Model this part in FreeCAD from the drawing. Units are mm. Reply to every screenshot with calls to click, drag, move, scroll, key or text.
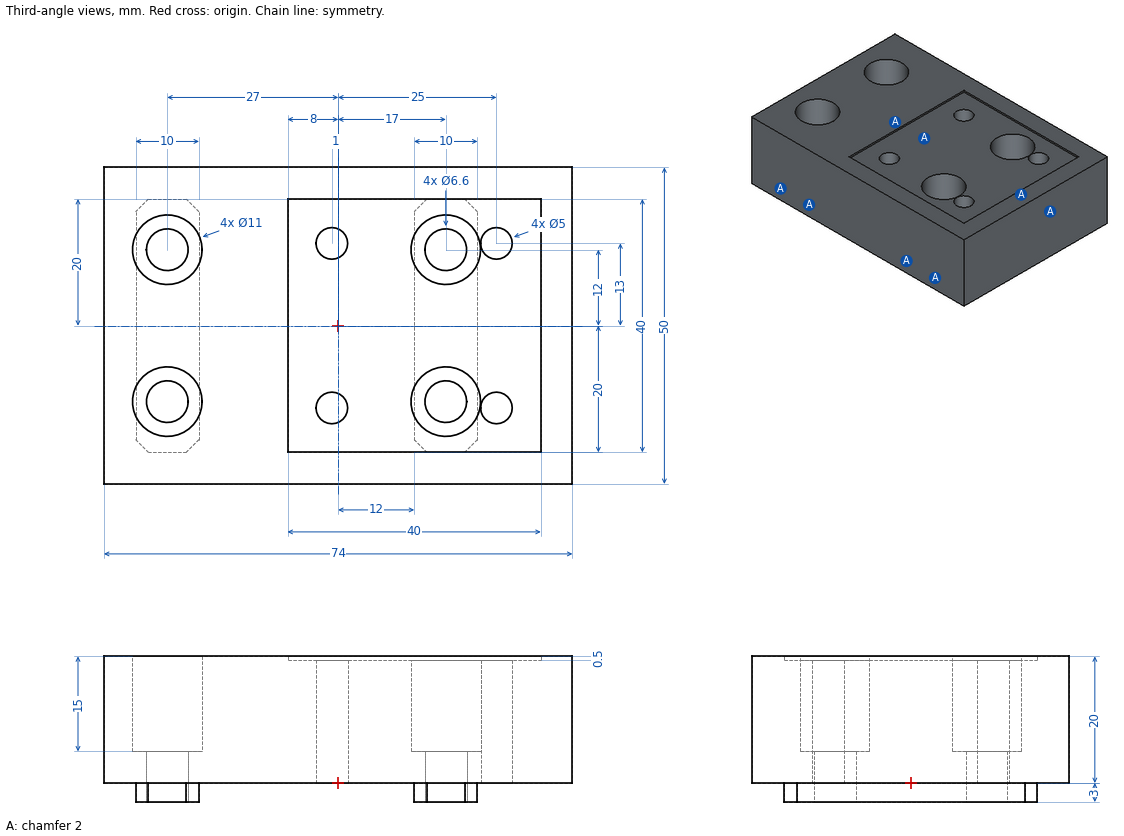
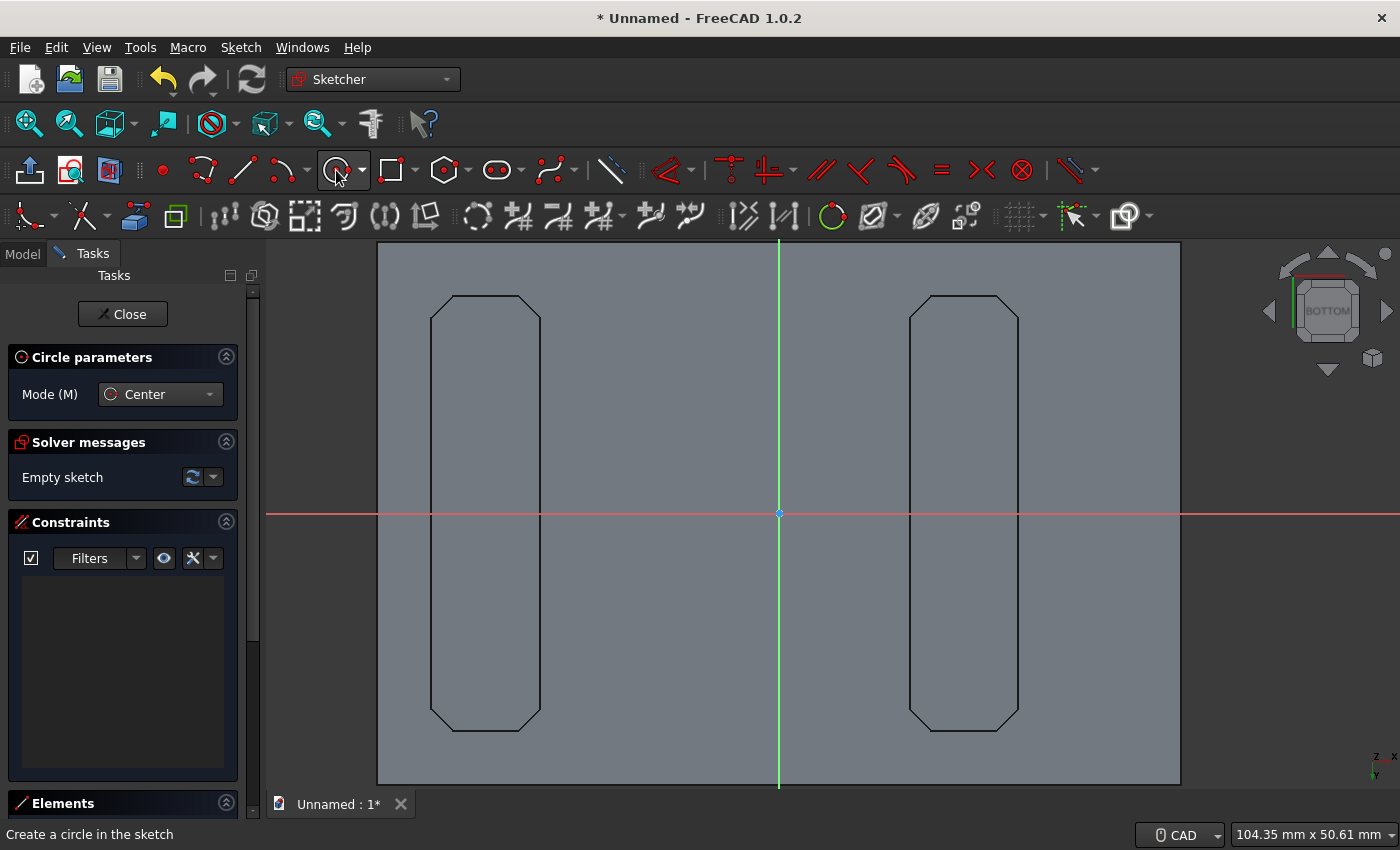
click(964, 644)
move(989, 619)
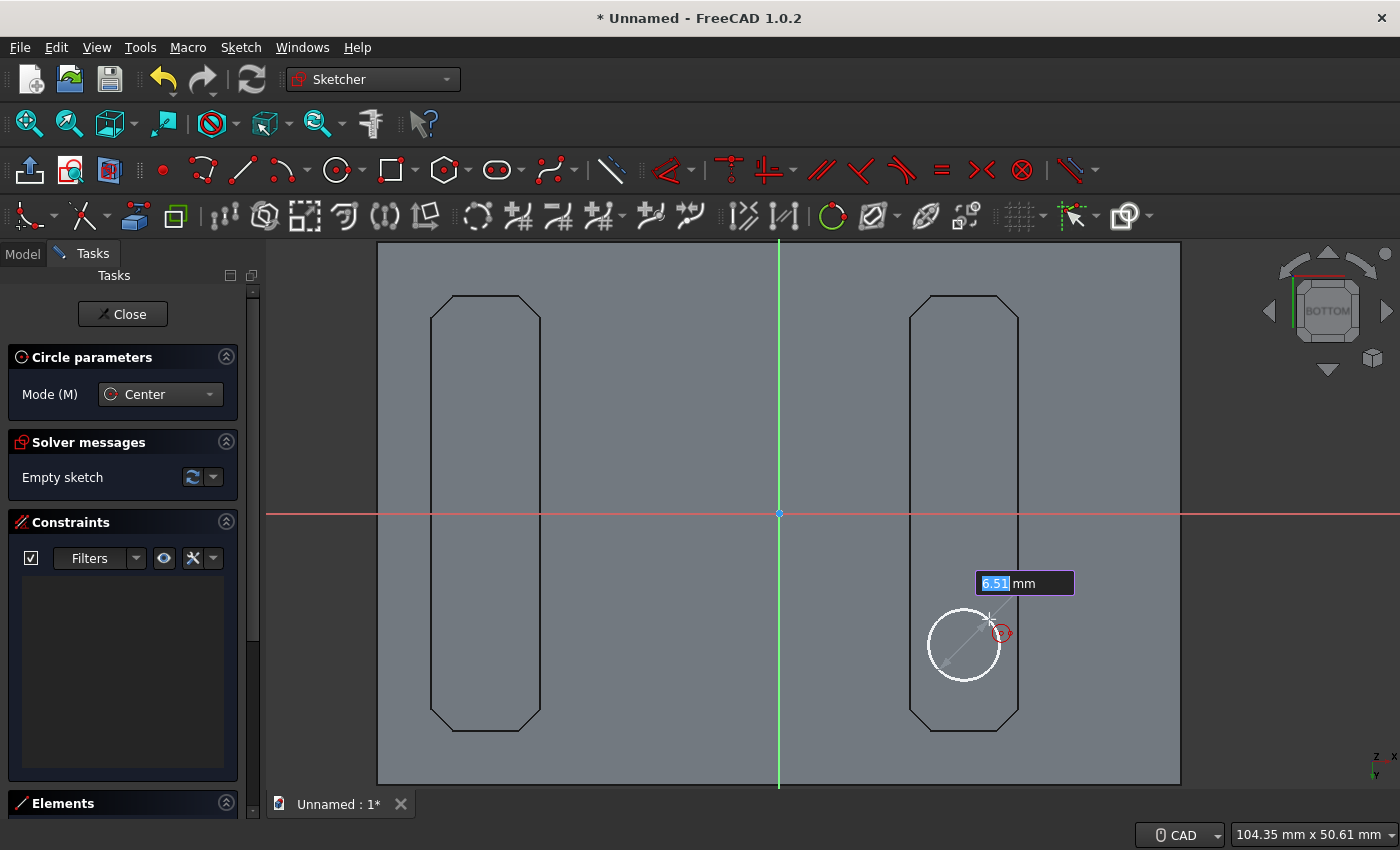
text(6.6)
key(Return)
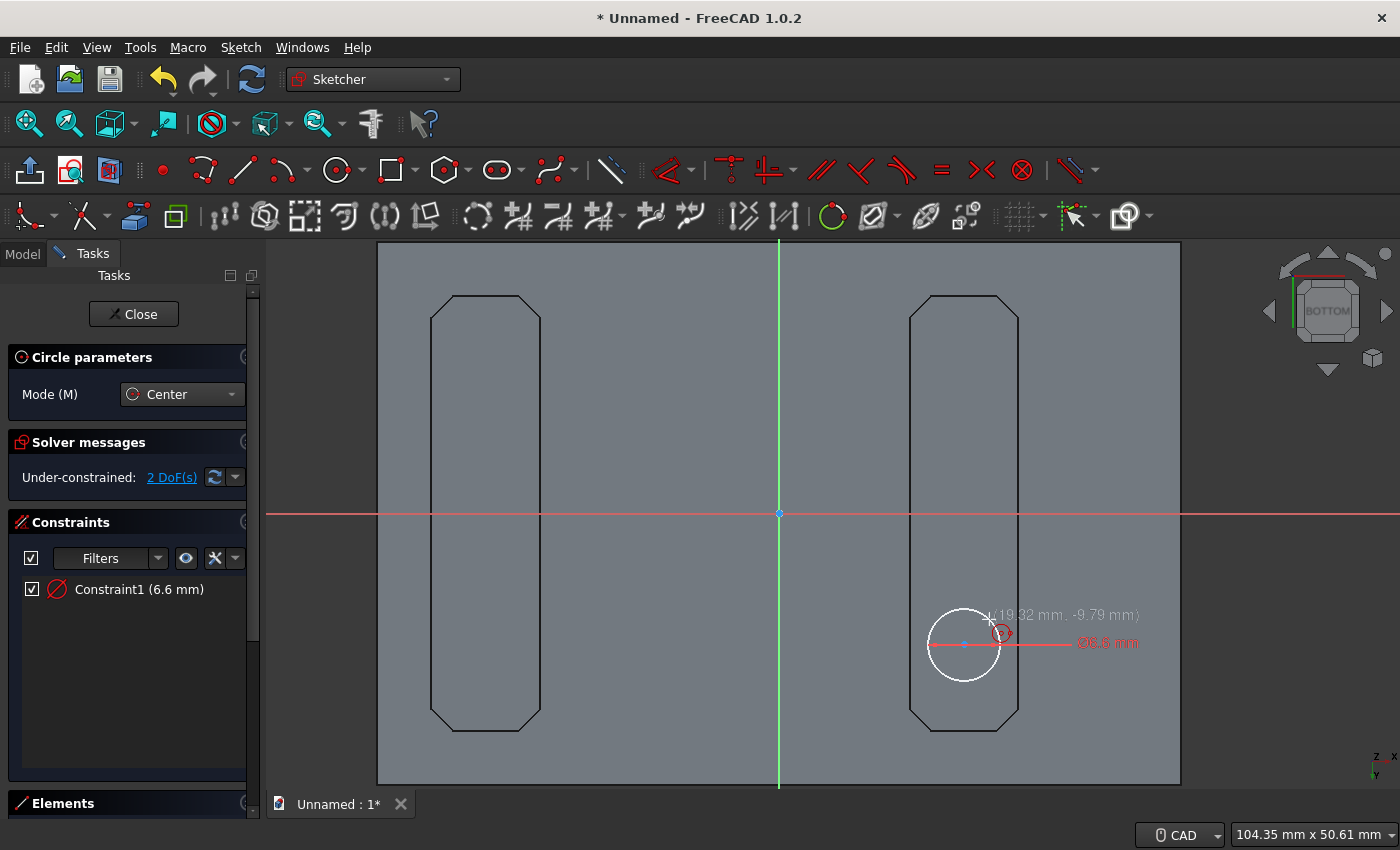
click(486, 644)
move(511, 619)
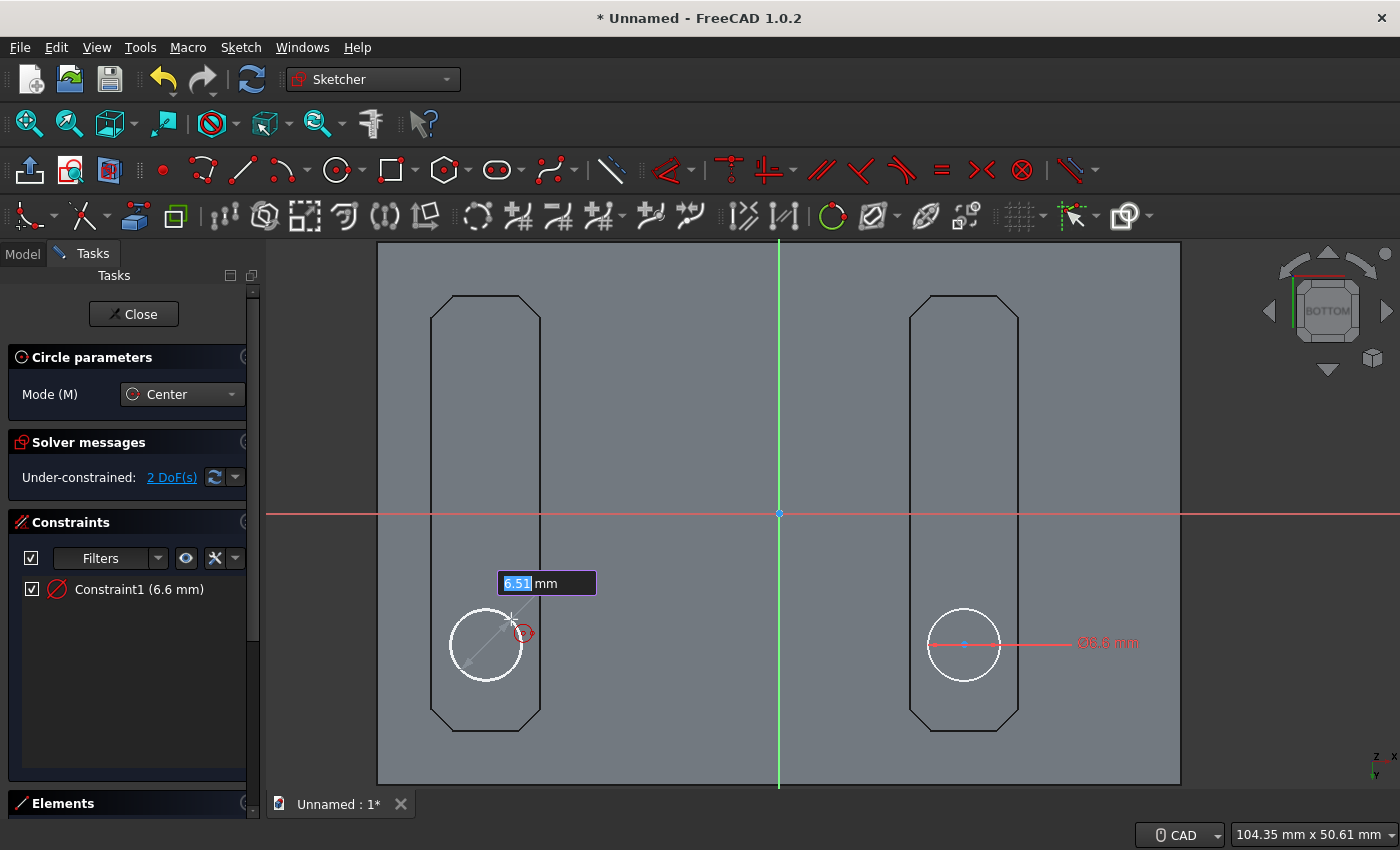
text(6.6)
key(Return)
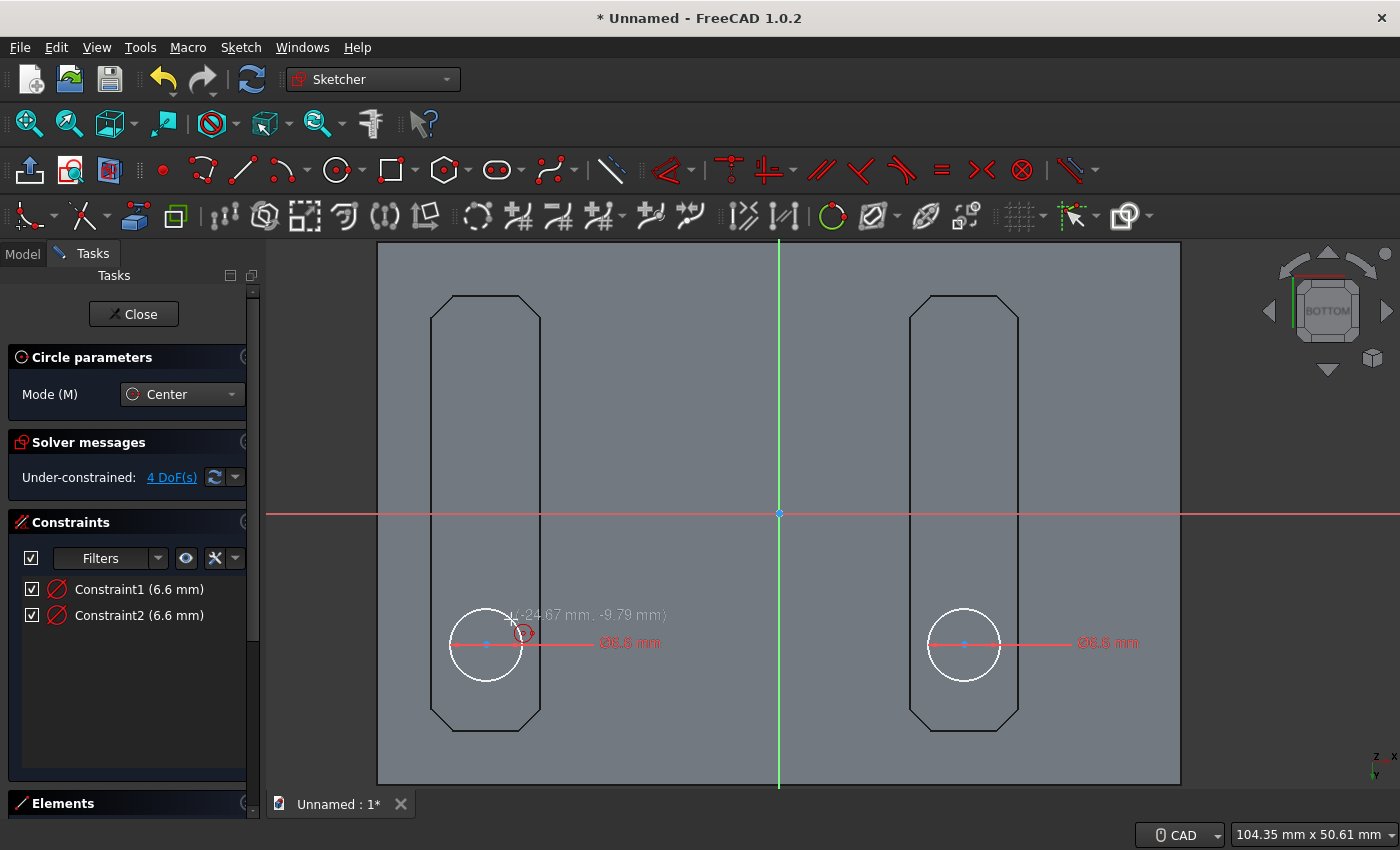
click(1051, 655)
move(1070, 636)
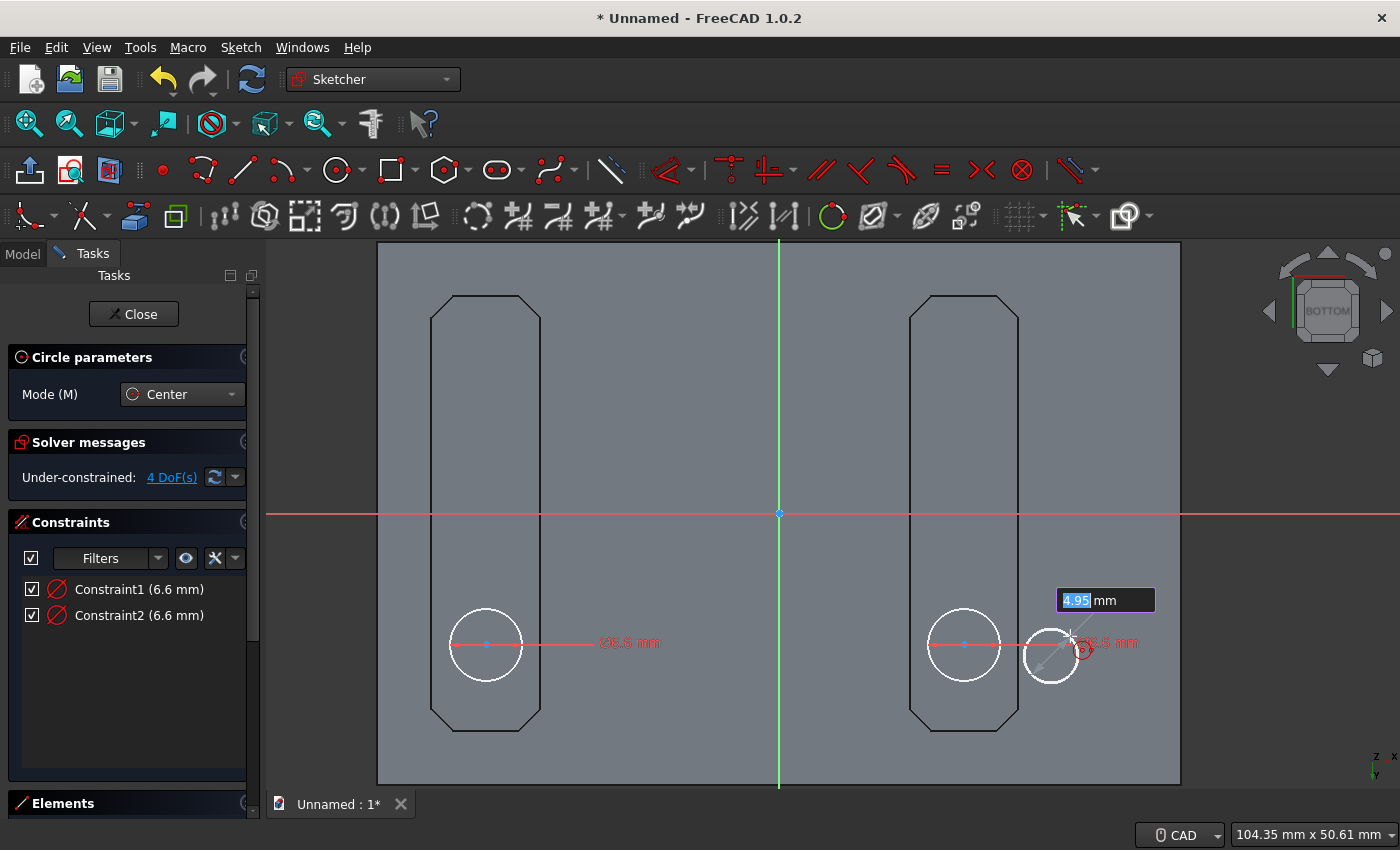
text(5)
key(Return)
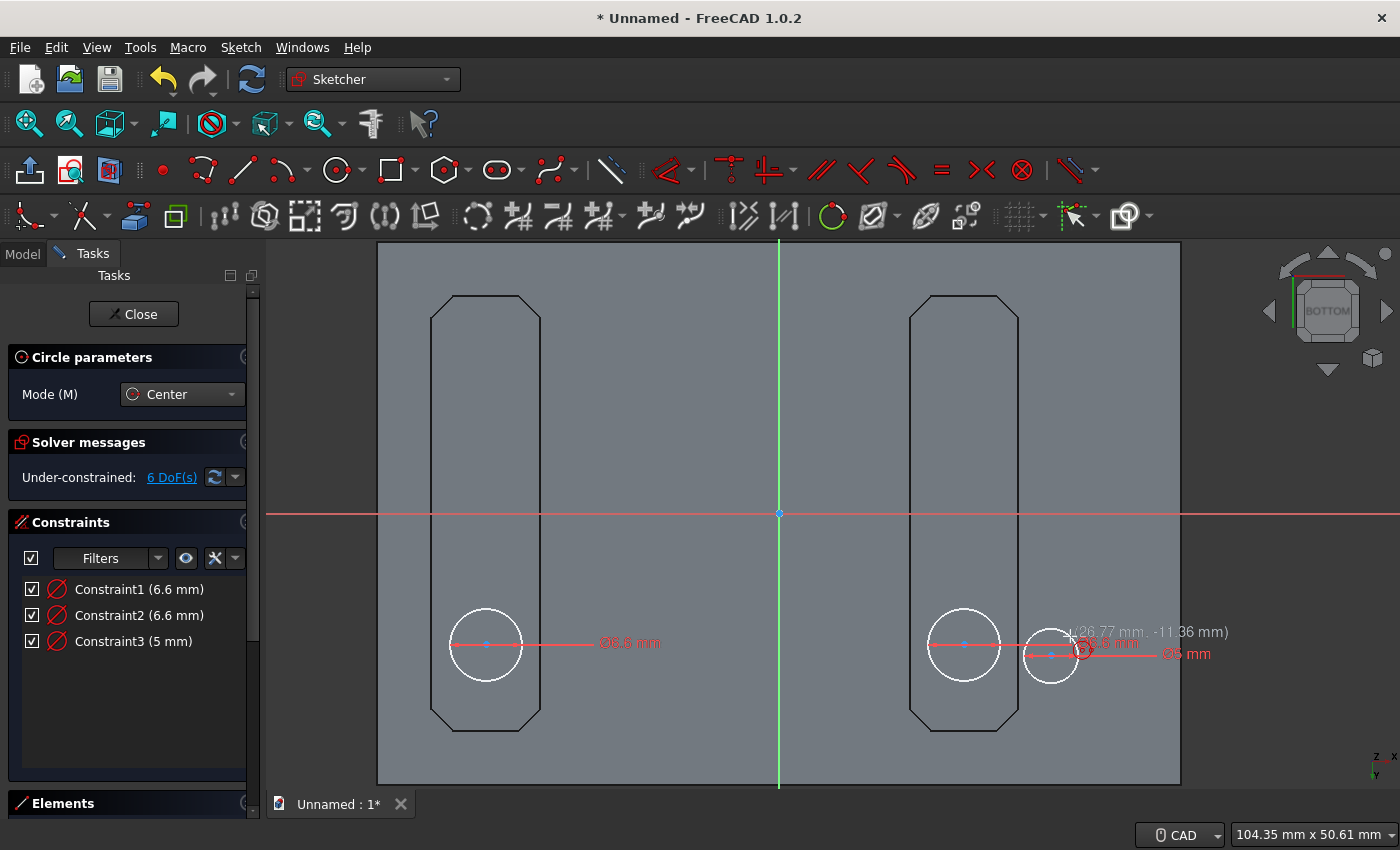
scroll(768, 655, up, 2)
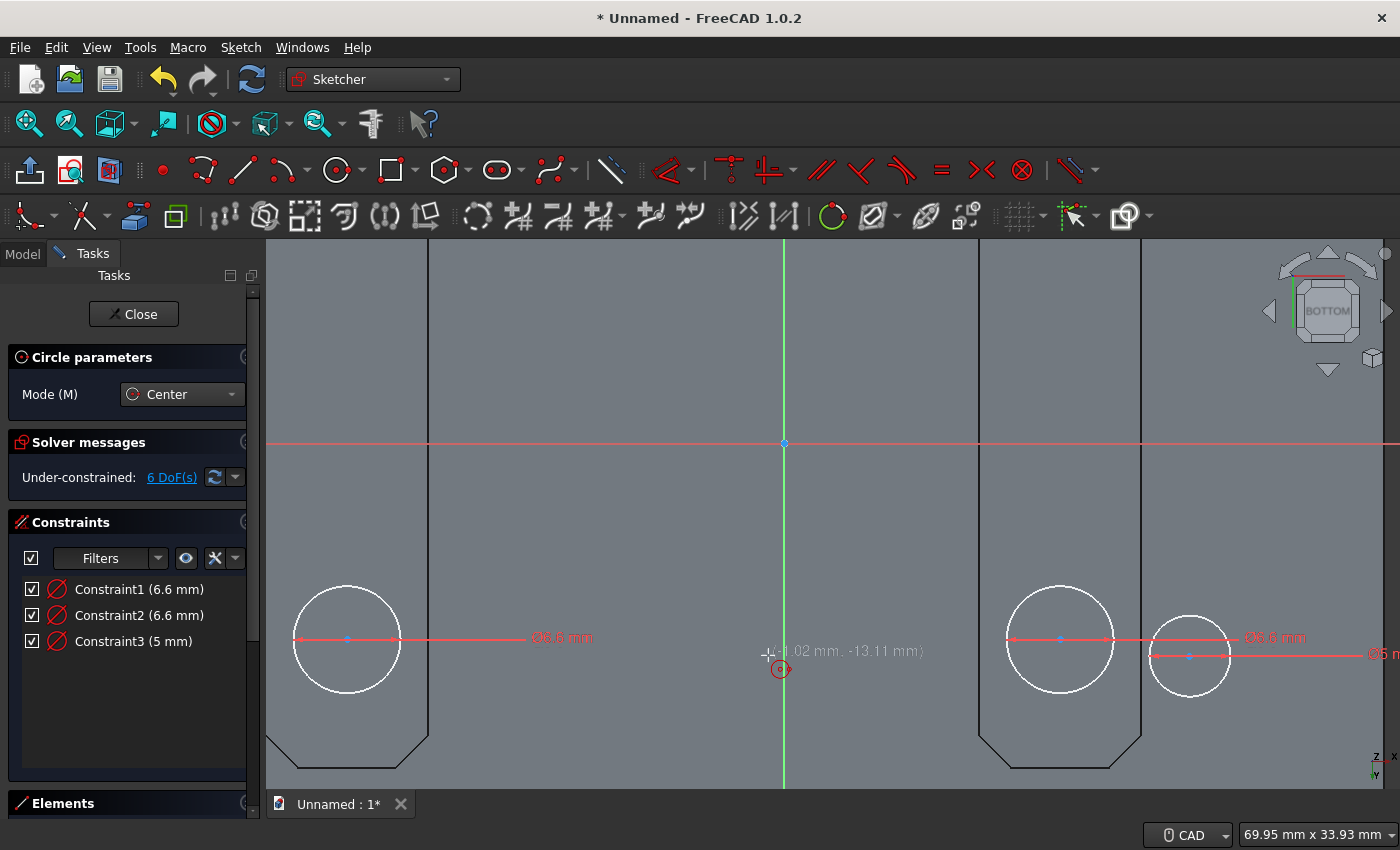
click(768, 654)
move(739, 626)